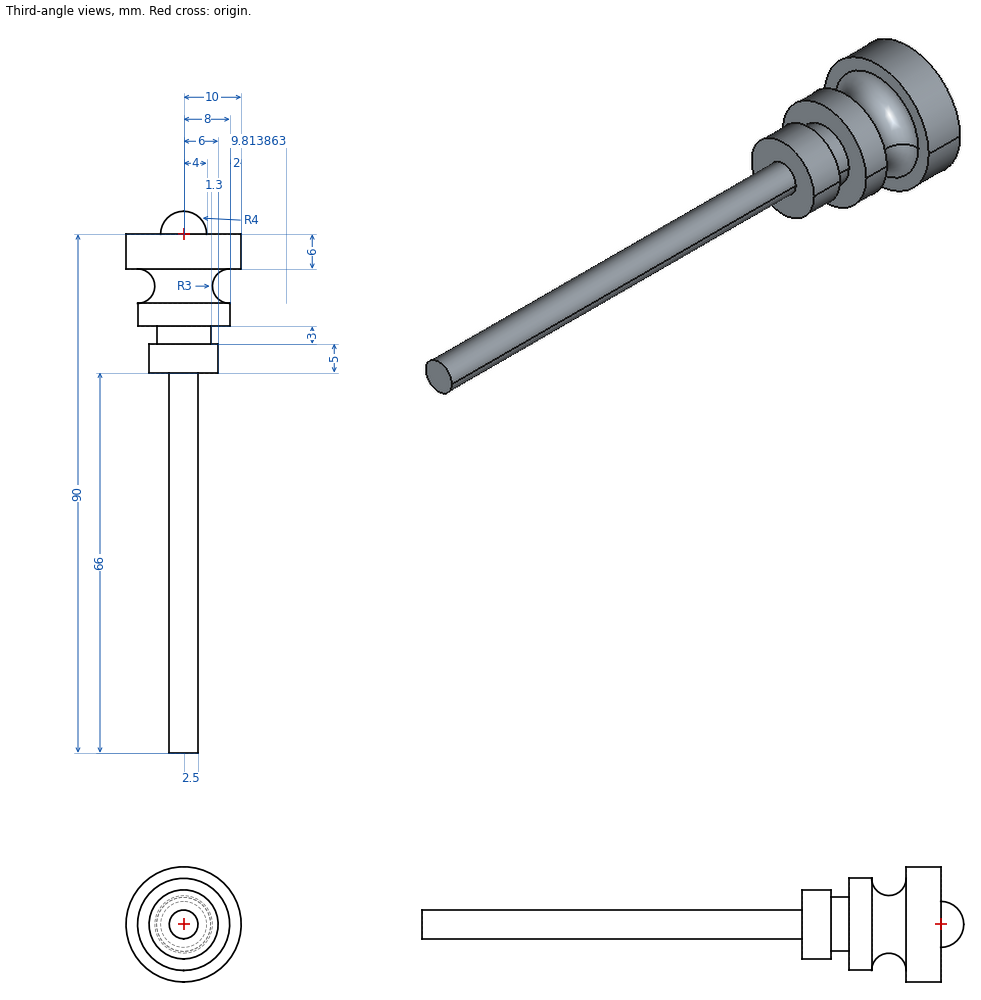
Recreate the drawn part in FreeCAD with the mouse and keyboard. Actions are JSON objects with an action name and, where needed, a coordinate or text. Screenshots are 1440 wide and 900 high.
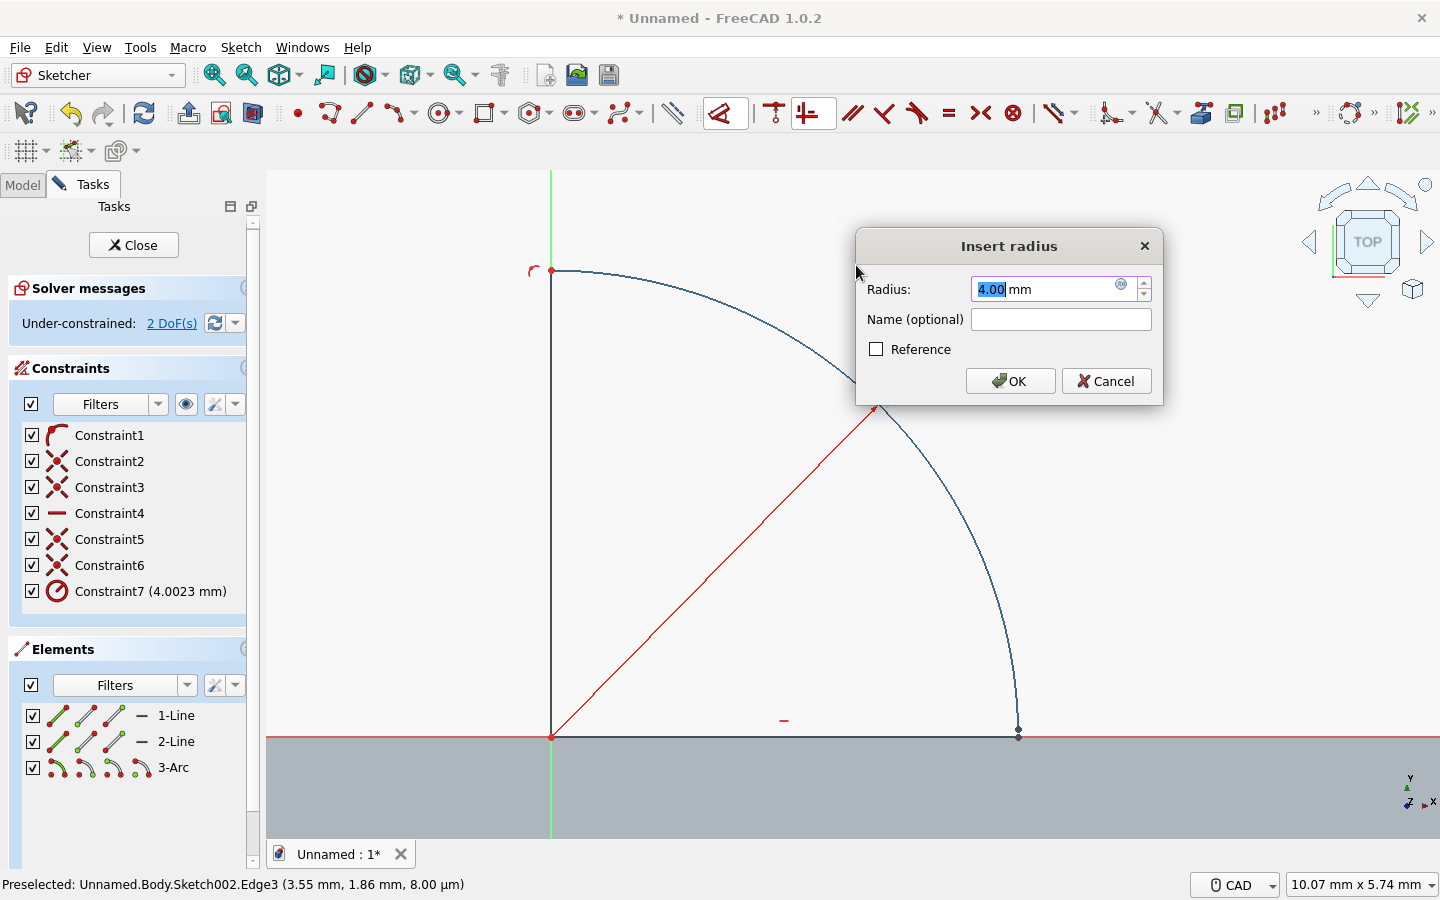
{"action": "type", "text": "4"}
{"action": "key", "text": "Return"}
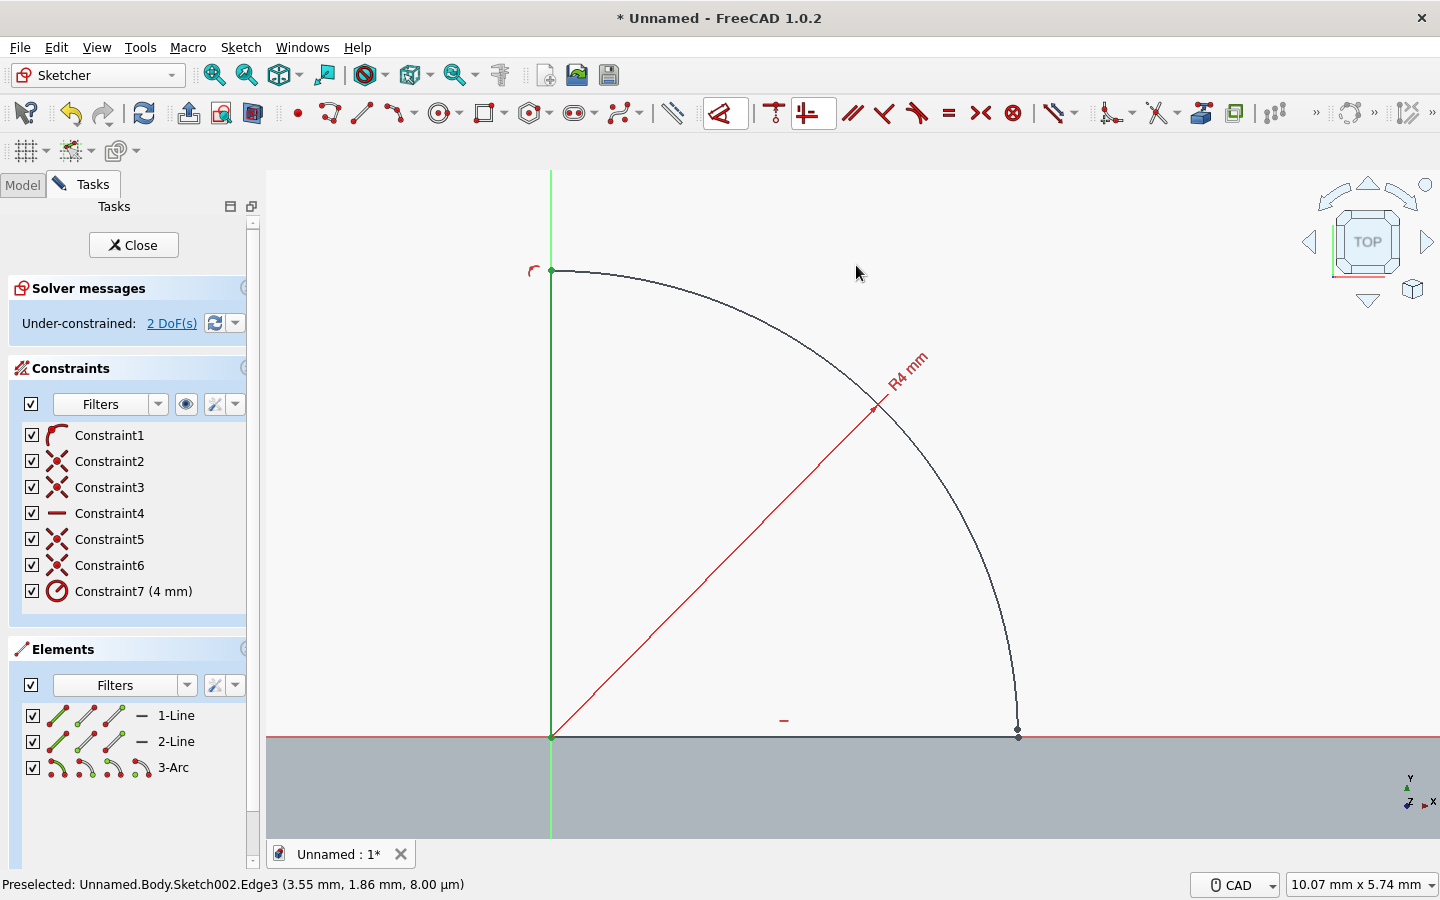
{"action": "left_click", "coordinate": [1018, 729]}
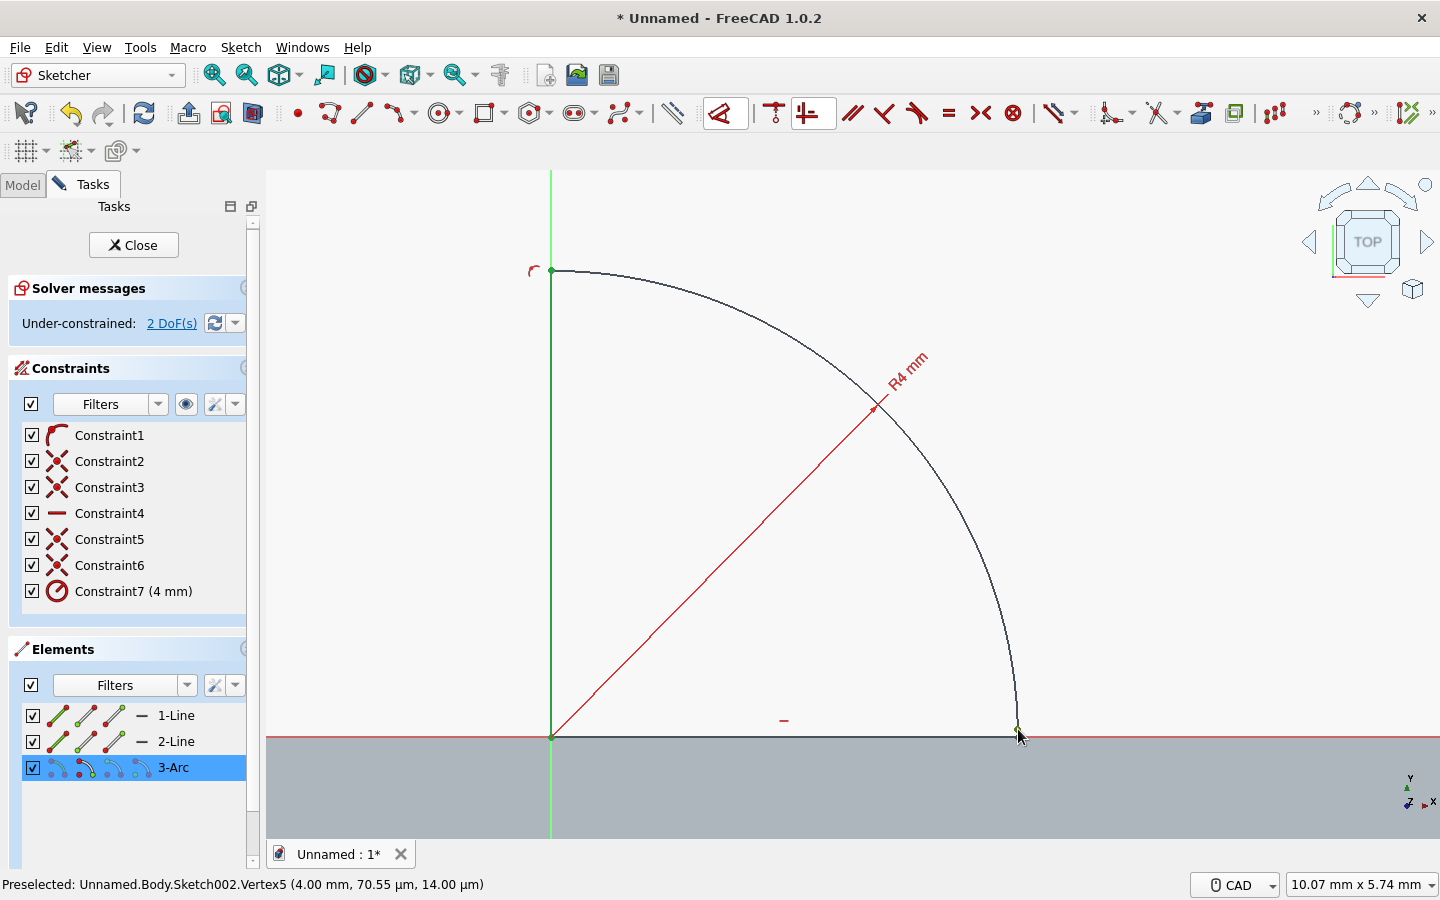
{"action": "left_click", "coordinate": [364, 737]}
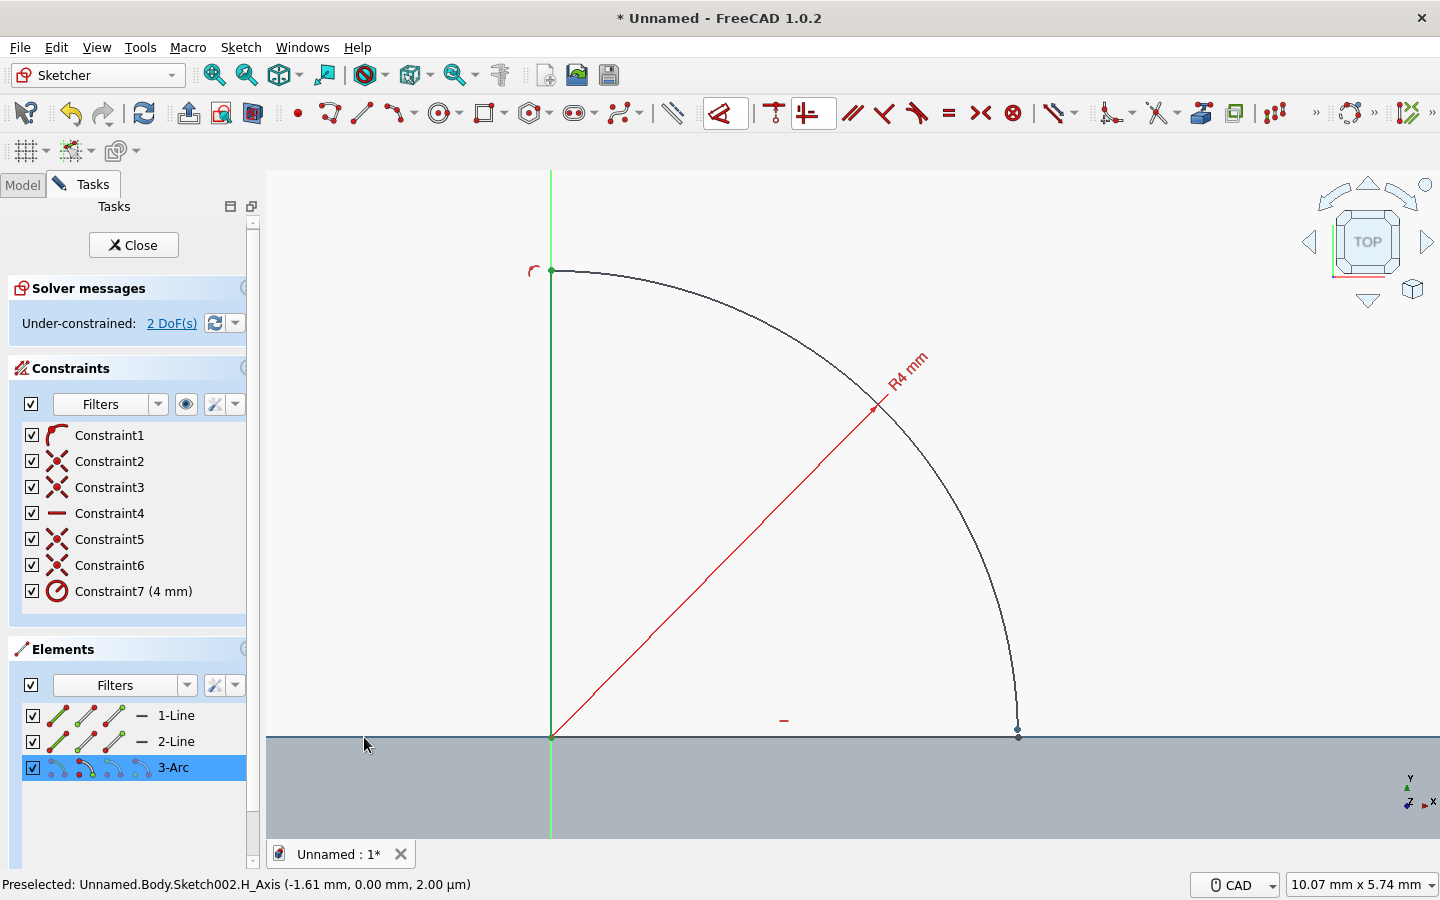
{"action": "key", "text": "c"}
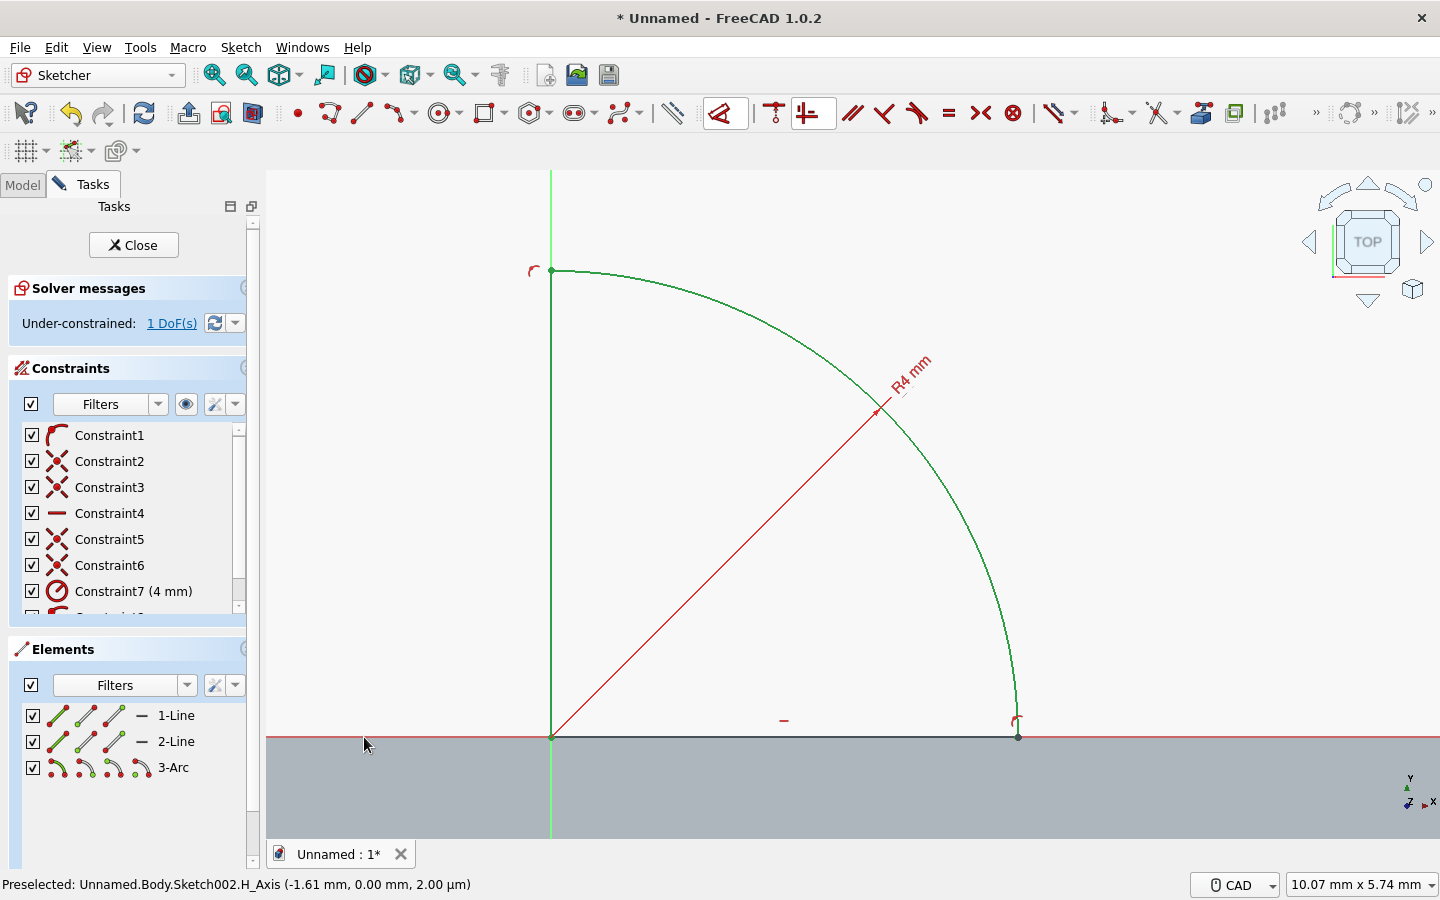
{"action": "left_click", "coordinate": [691, 737]}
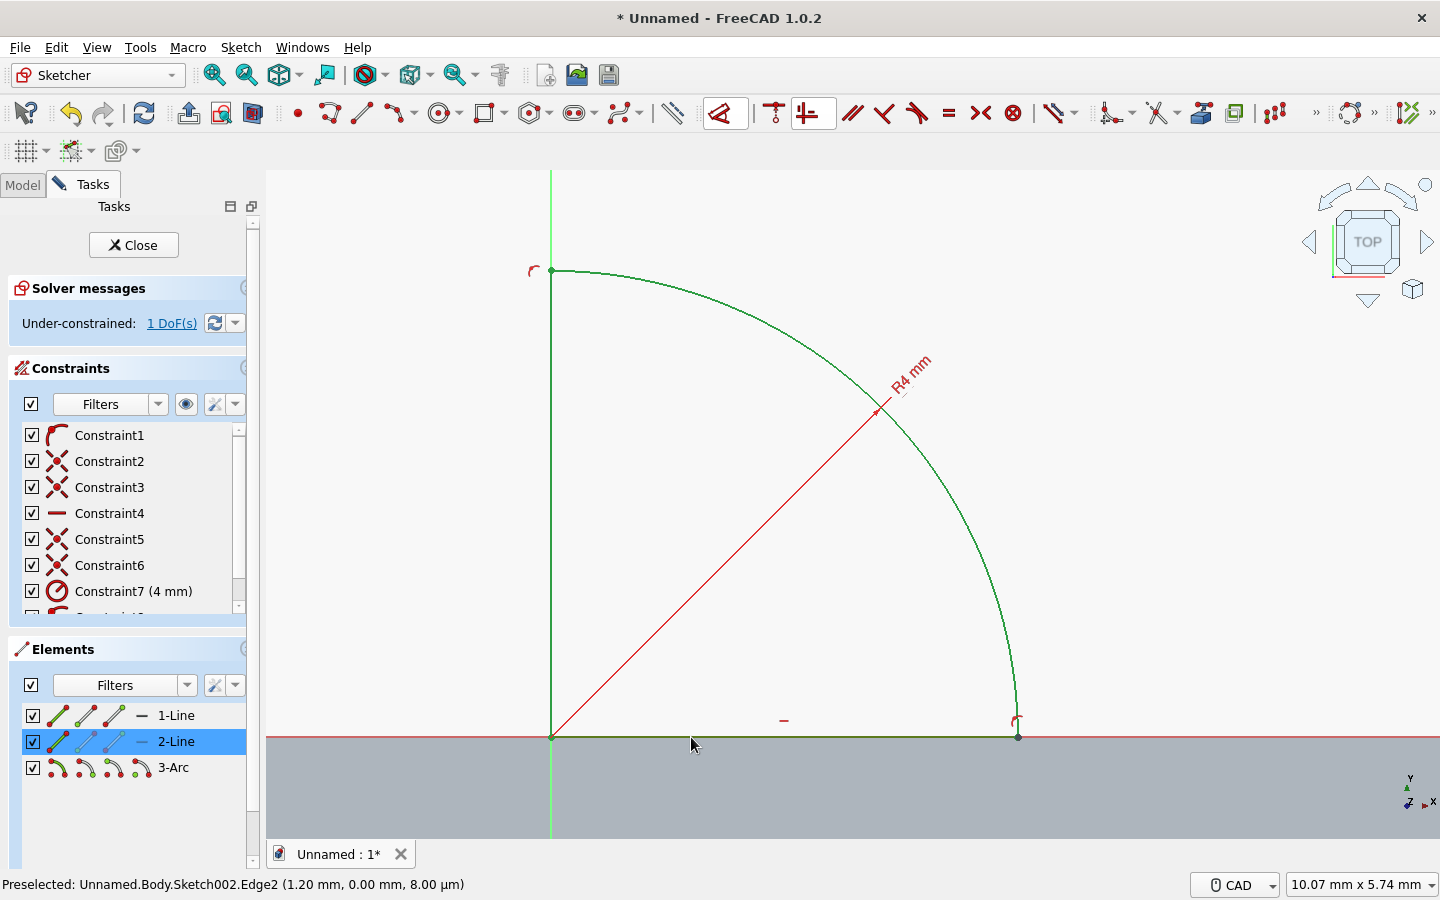
{"action": "key", "text": "l"}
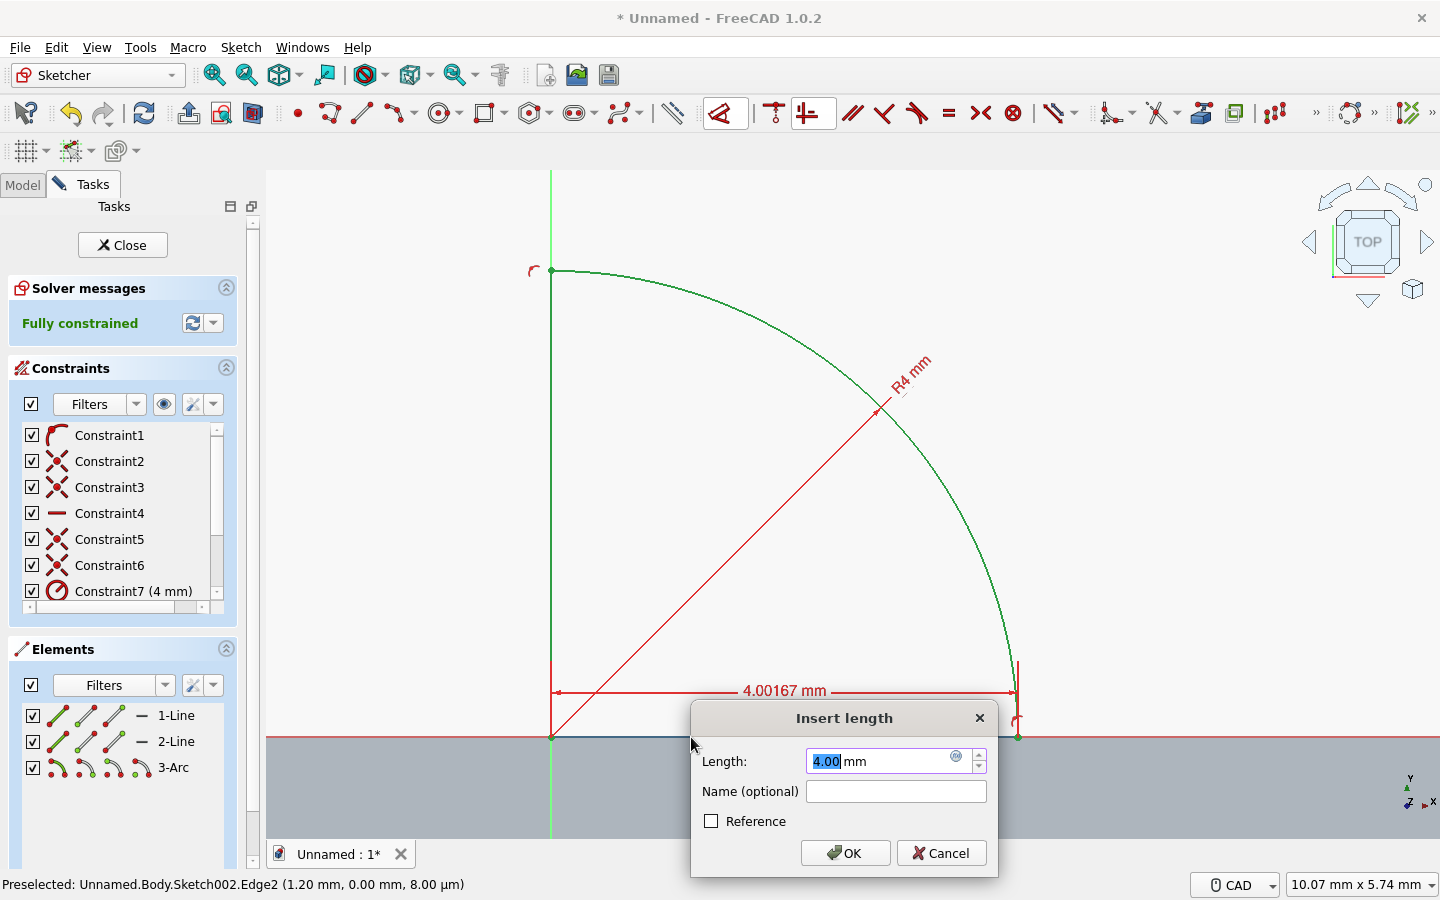
{"action": "type", "text": "4"}
{"action": "key", "text": "Return"}